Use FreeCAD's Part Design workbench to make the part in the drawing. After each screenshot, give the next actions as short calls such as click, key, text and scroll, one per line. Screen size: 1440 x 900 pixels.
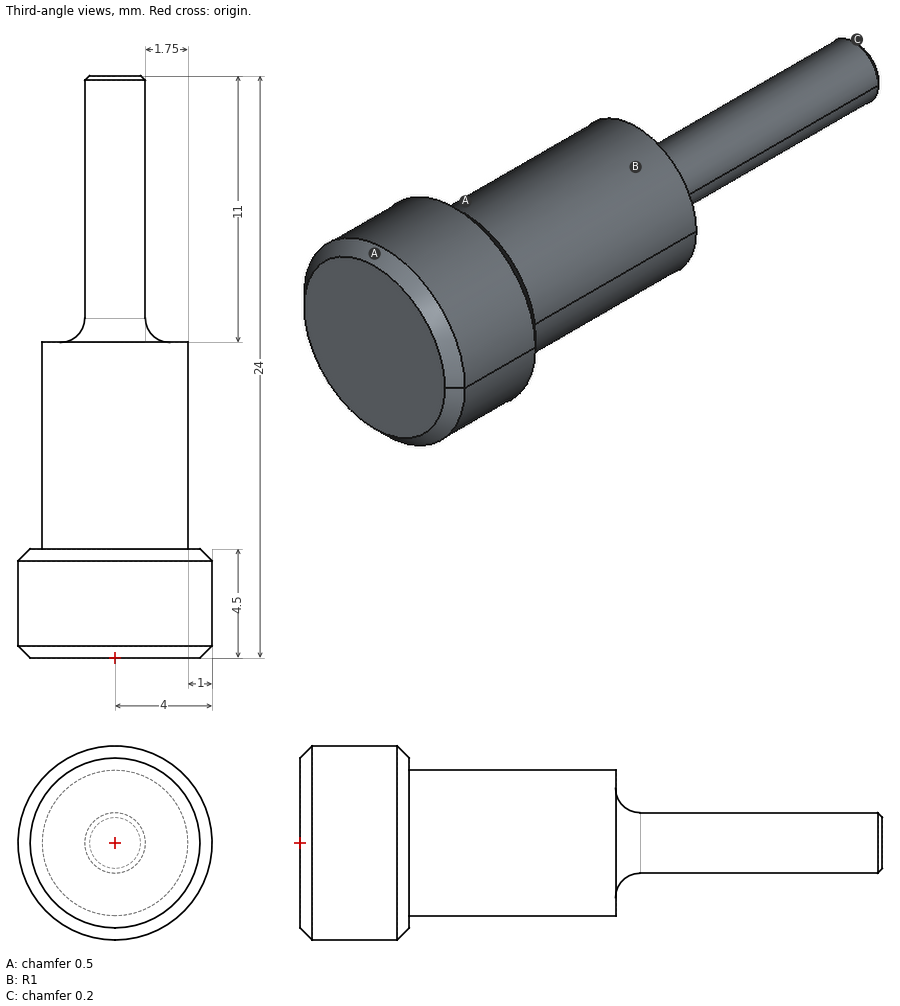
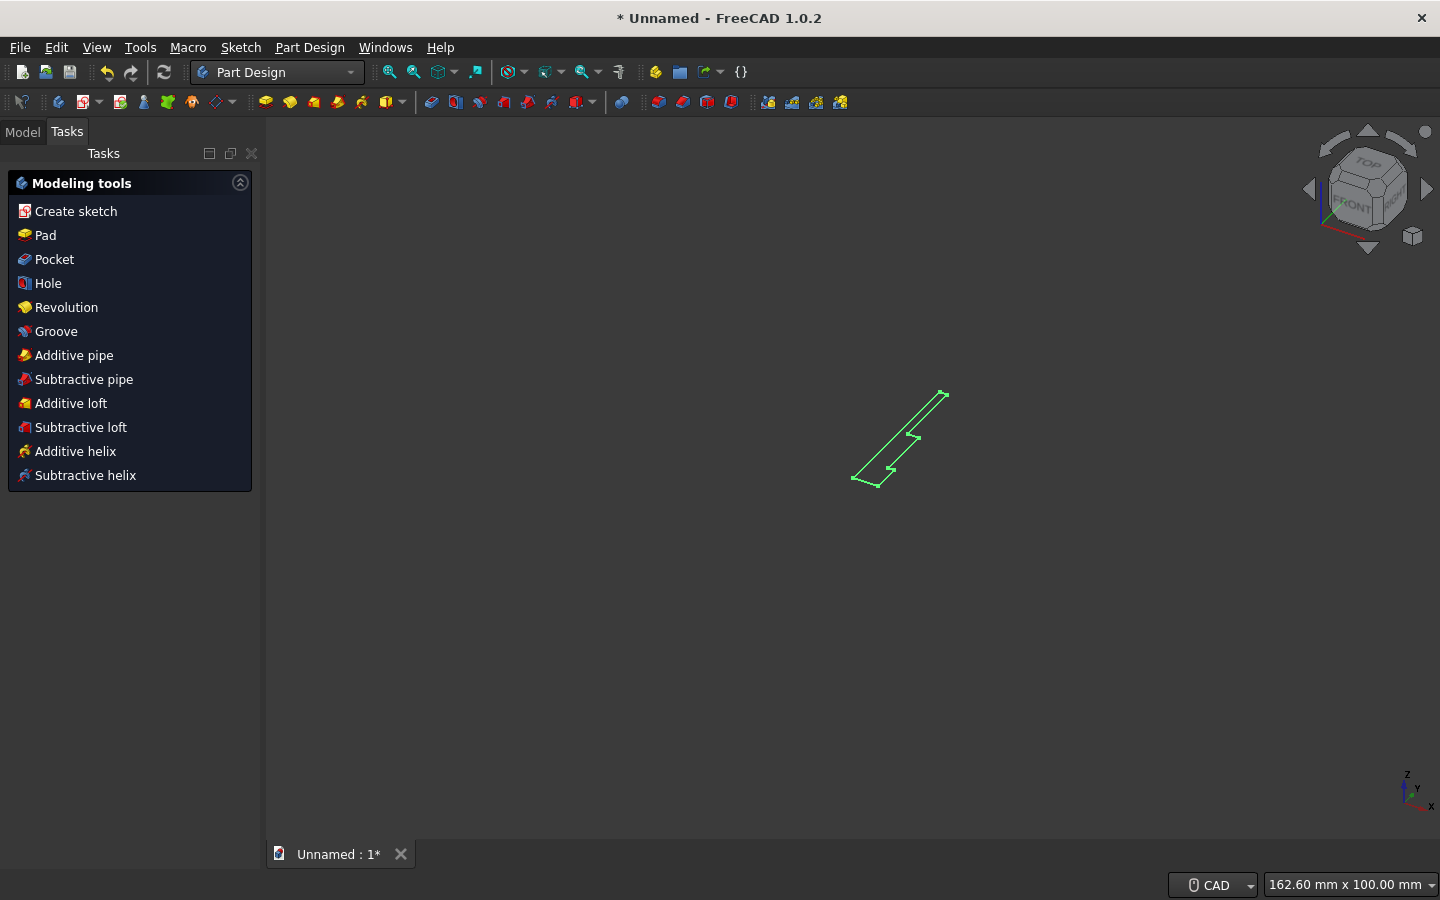
click(290, 102)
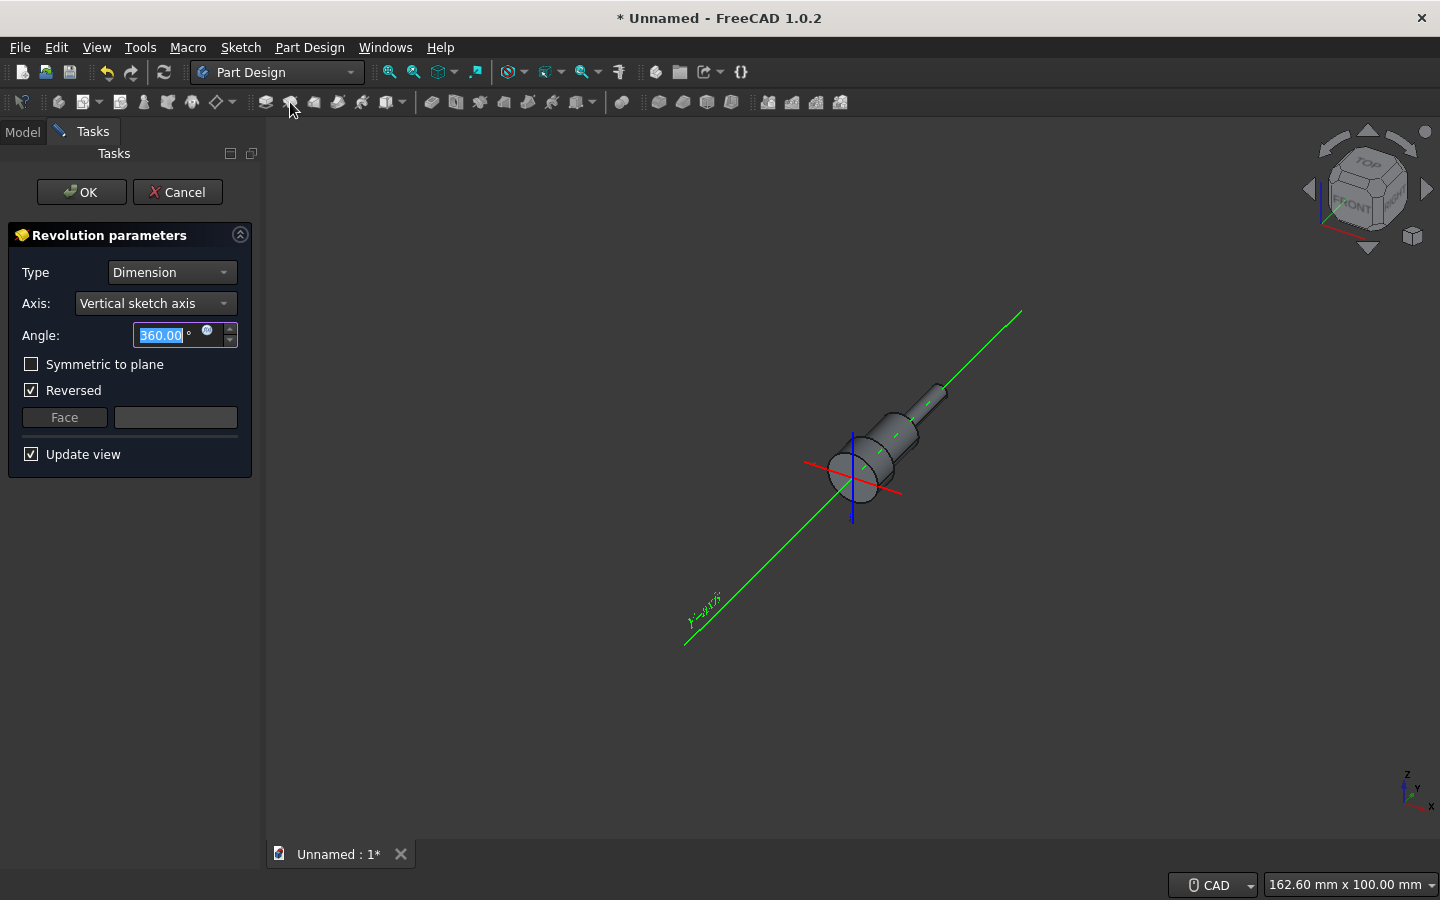
click(82, 192)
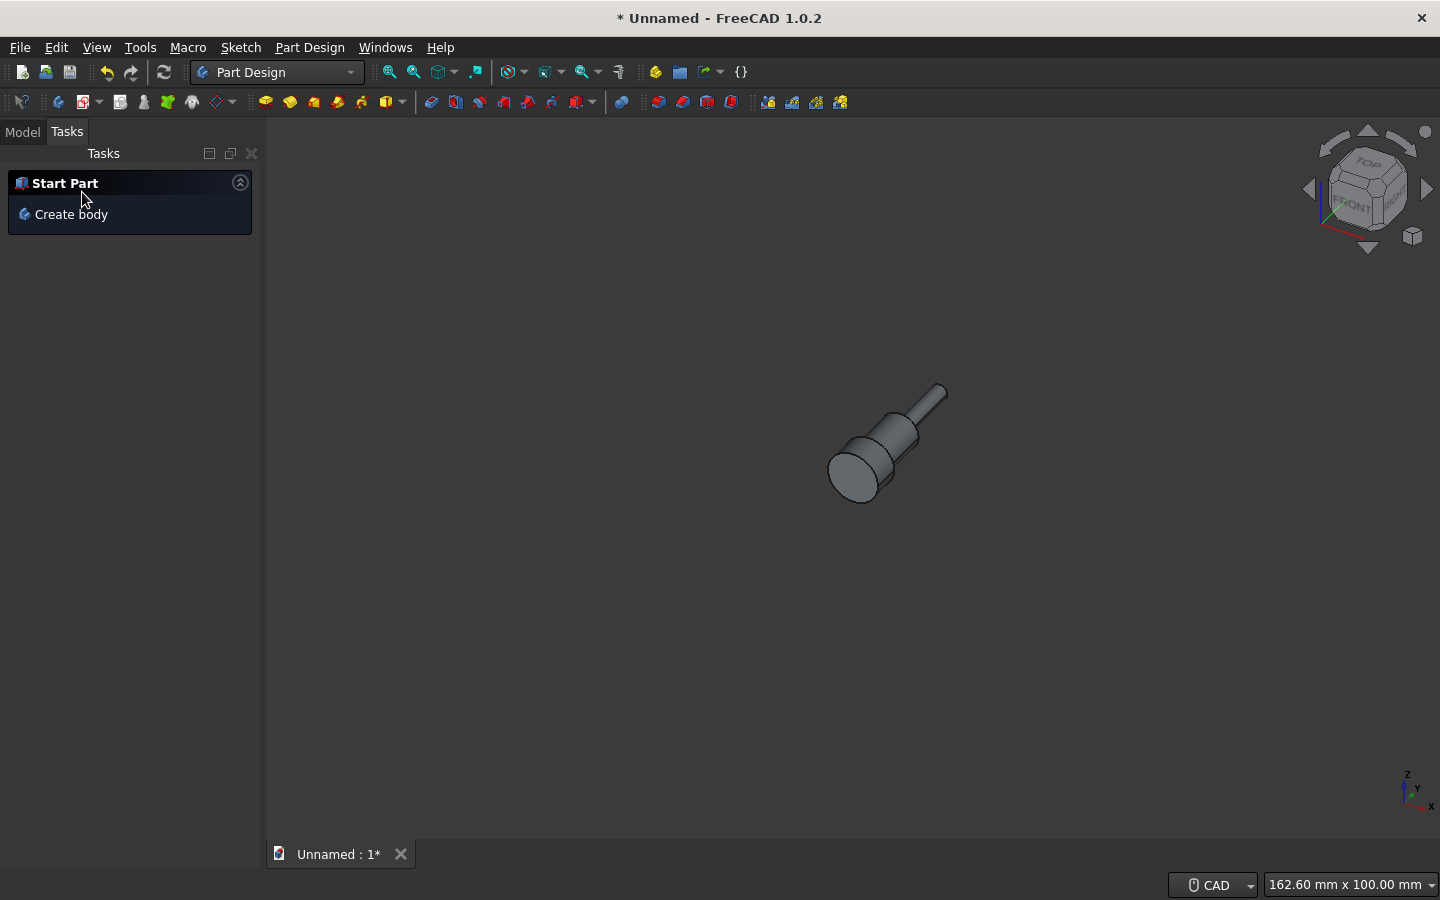
click(390, 72)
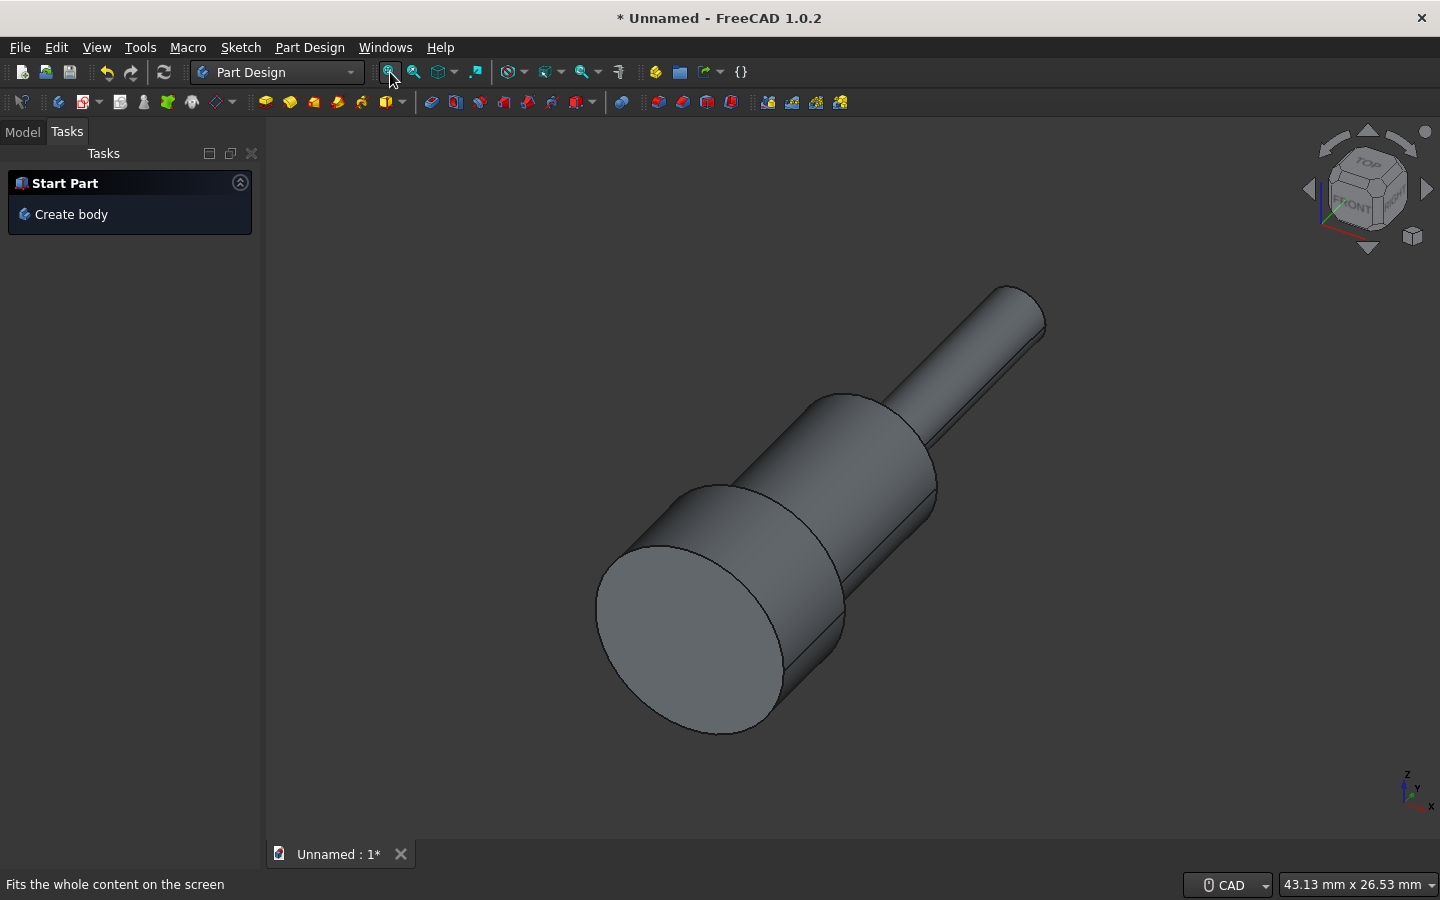
click(613, 562)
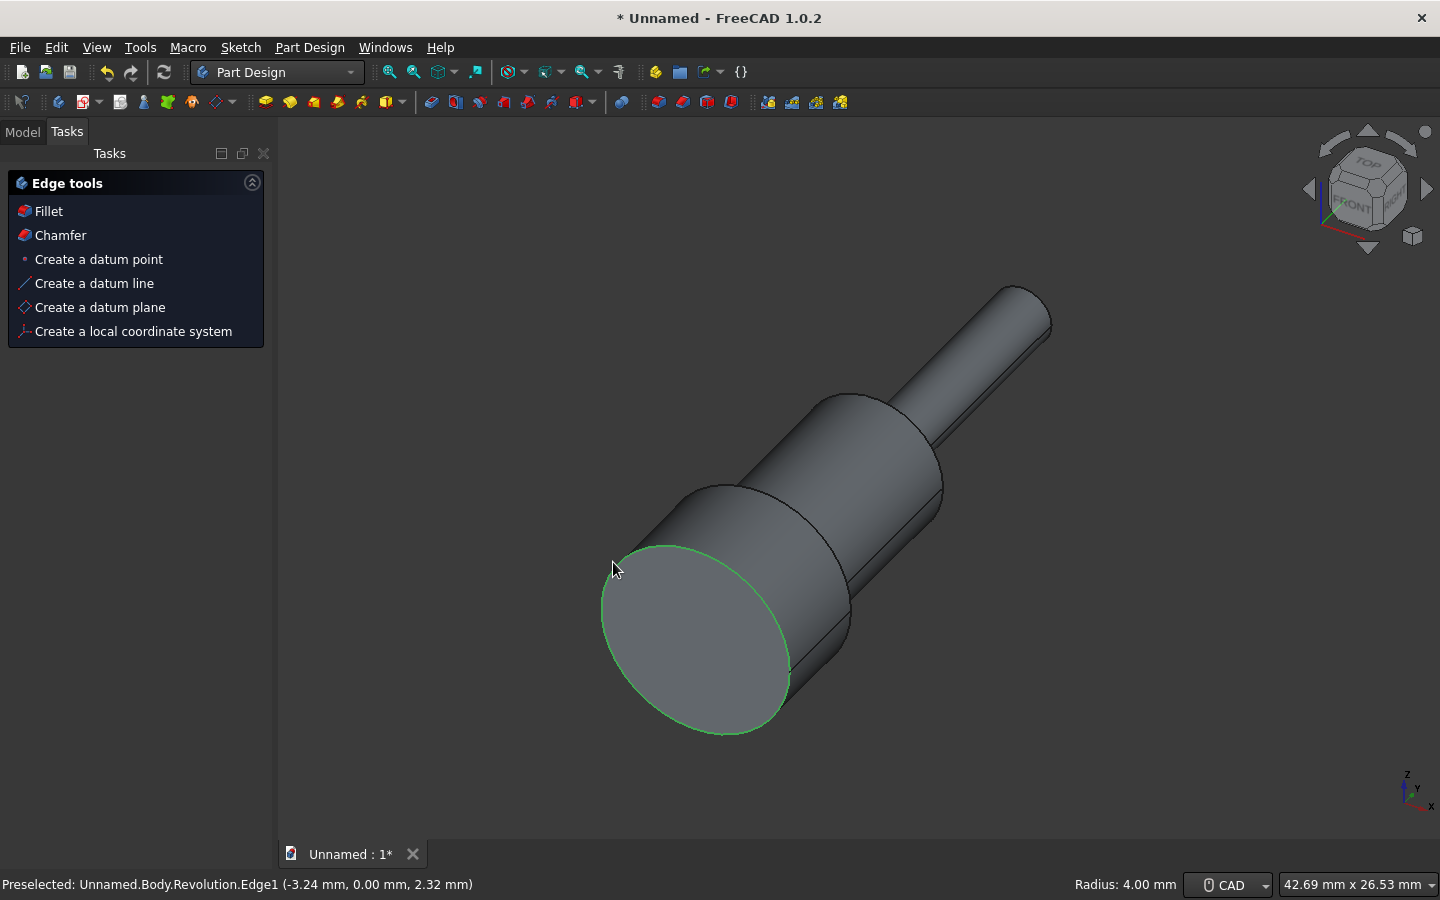
key(0)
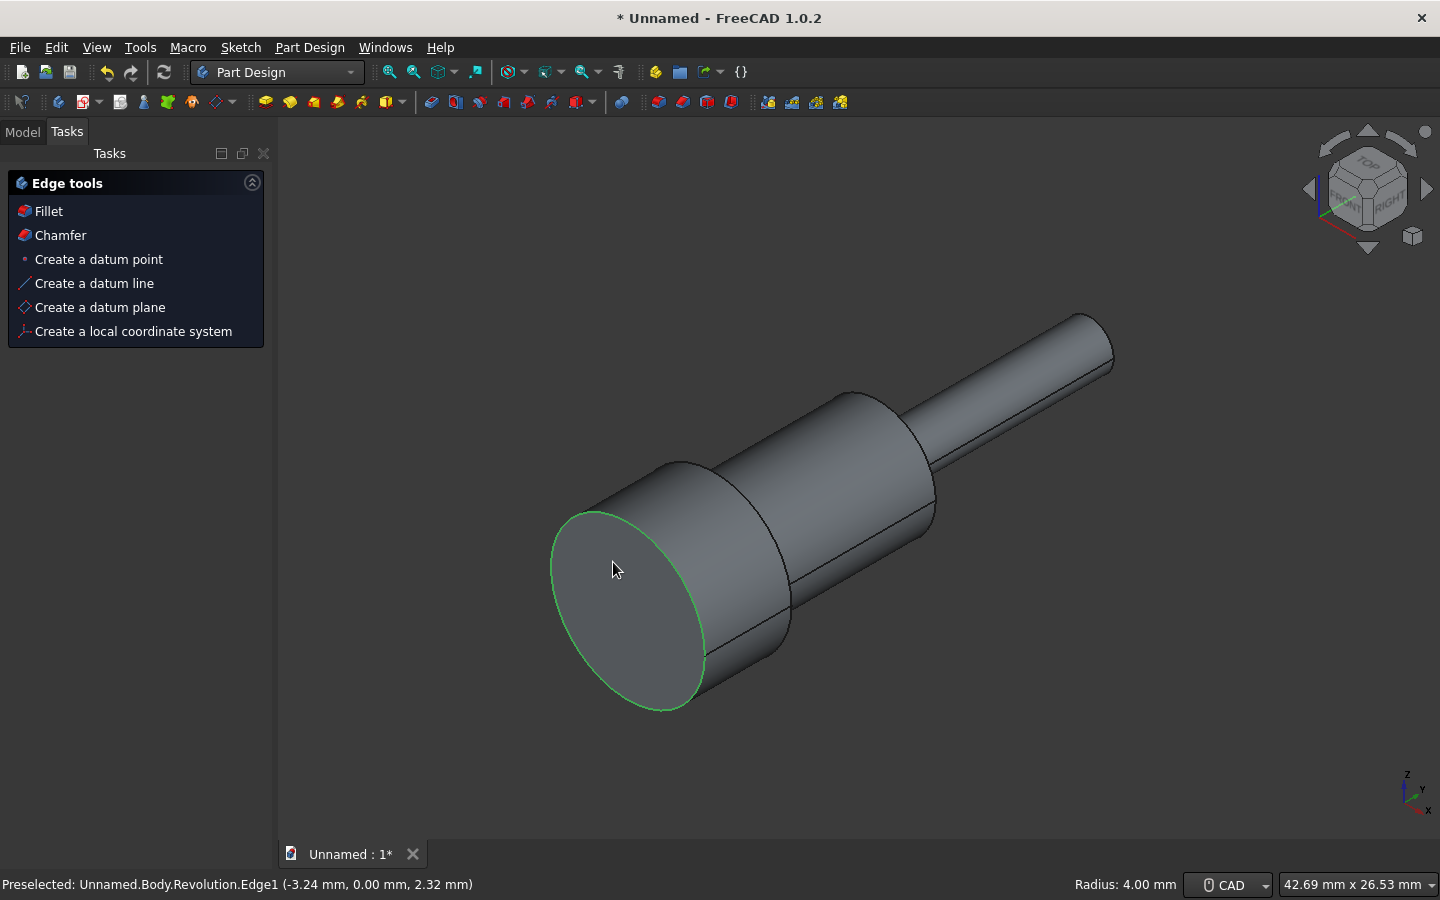
key(2)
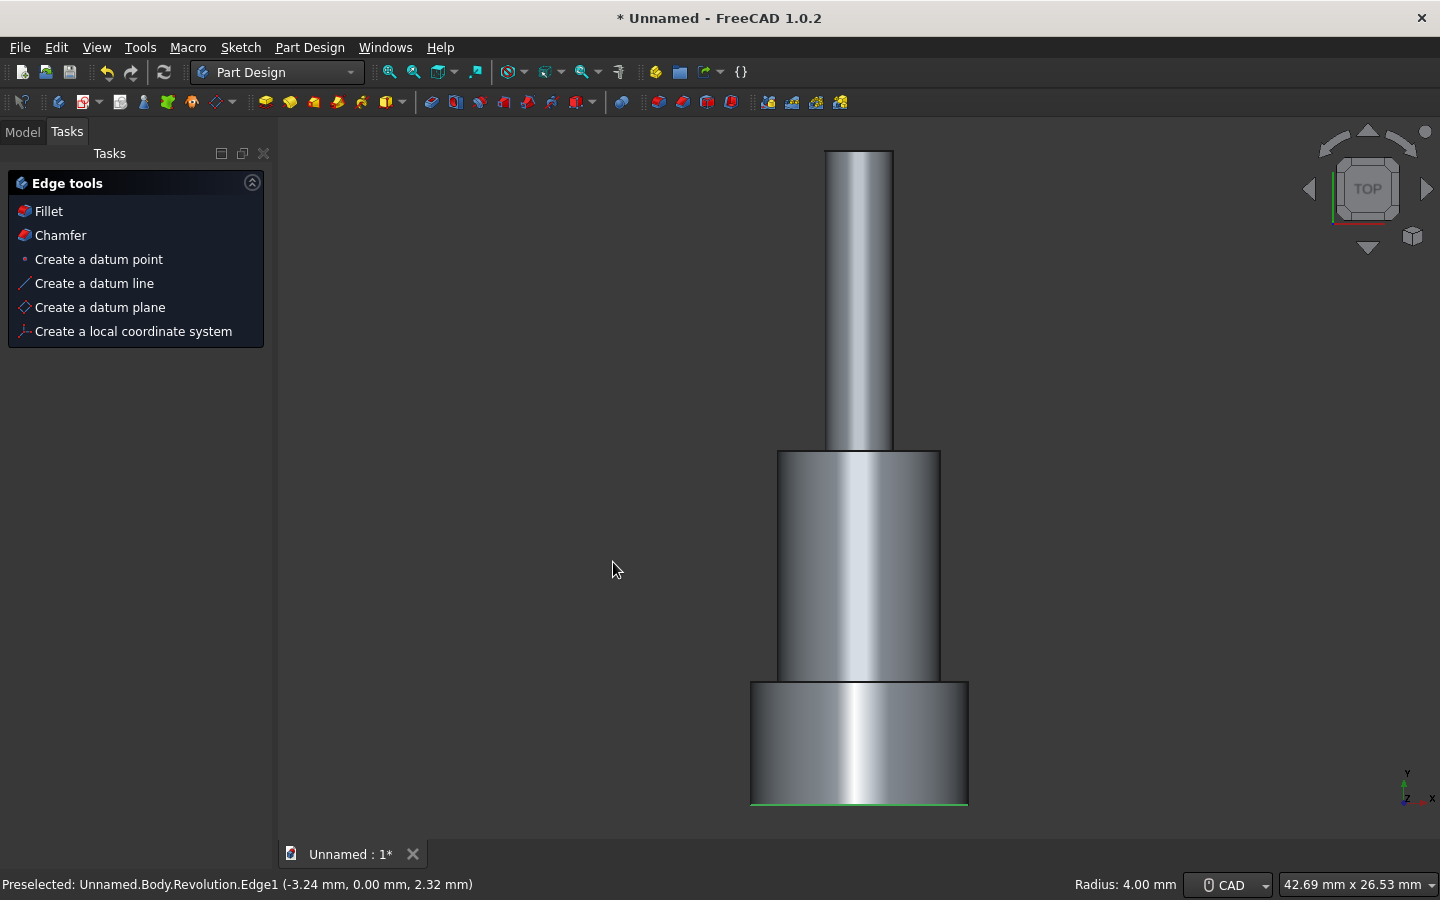
click(771, 681, ctrl)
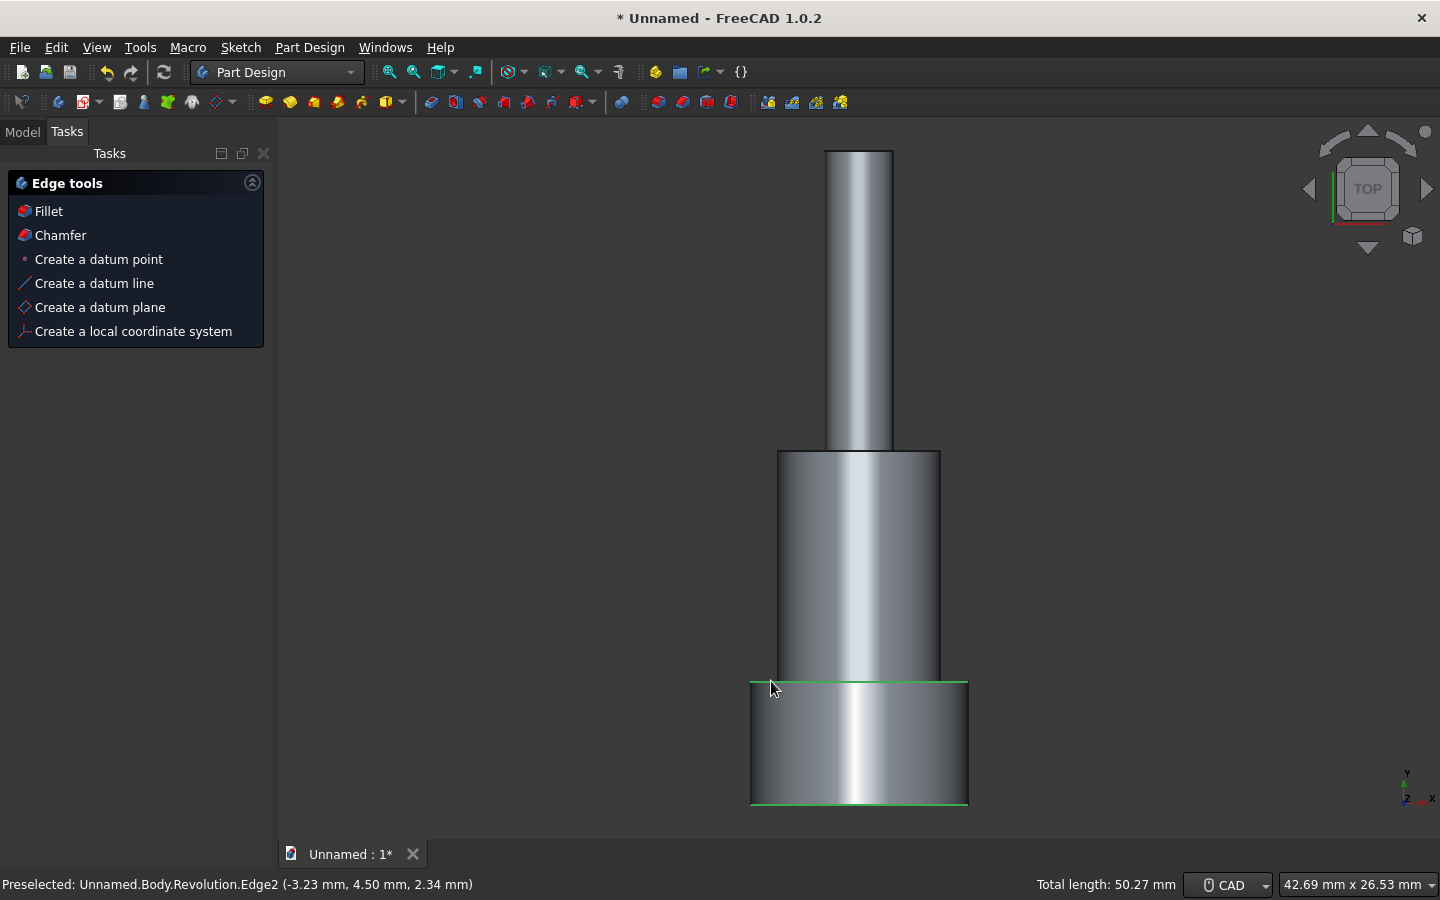
click(684, 102)